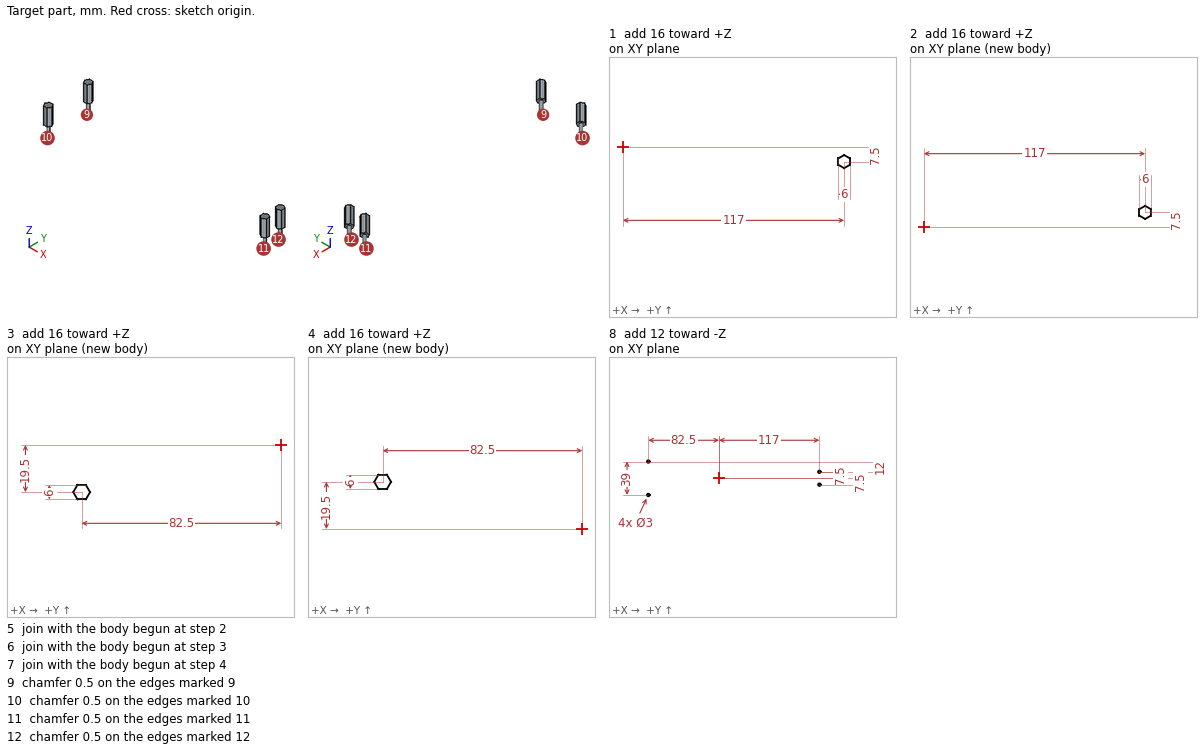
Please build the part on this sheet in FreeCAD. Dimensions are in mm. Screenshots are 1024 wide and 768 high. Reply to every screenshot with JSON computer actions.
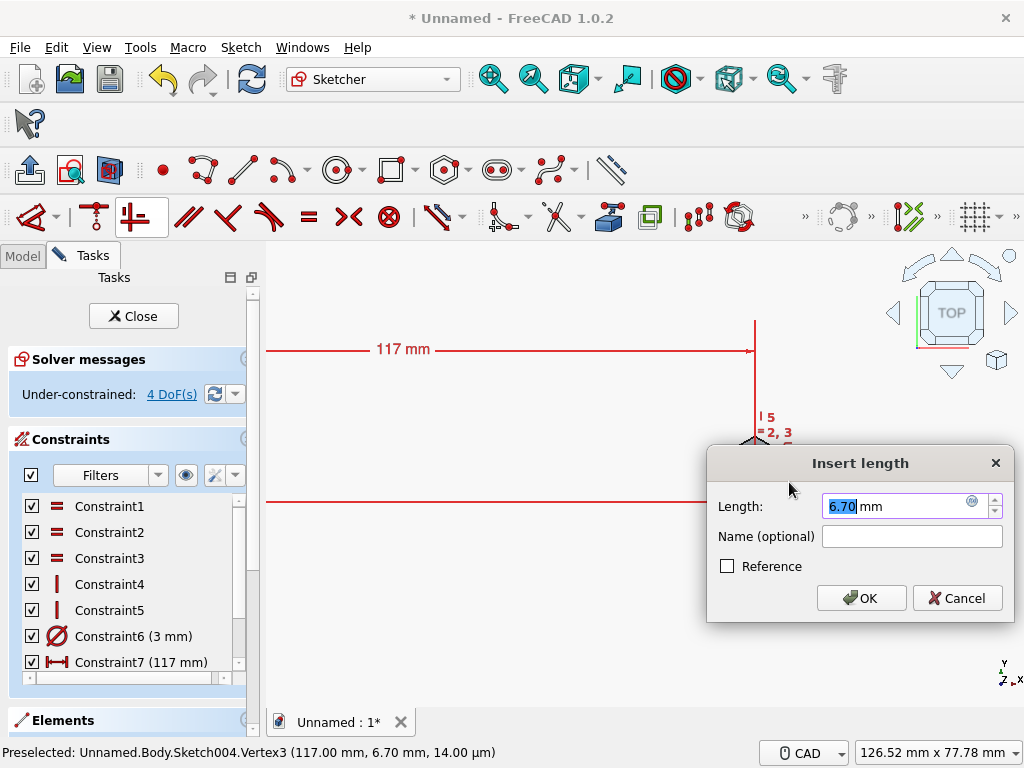
{"action": "type", "text": "7.5"}
{"action": "key", "text": "Return"}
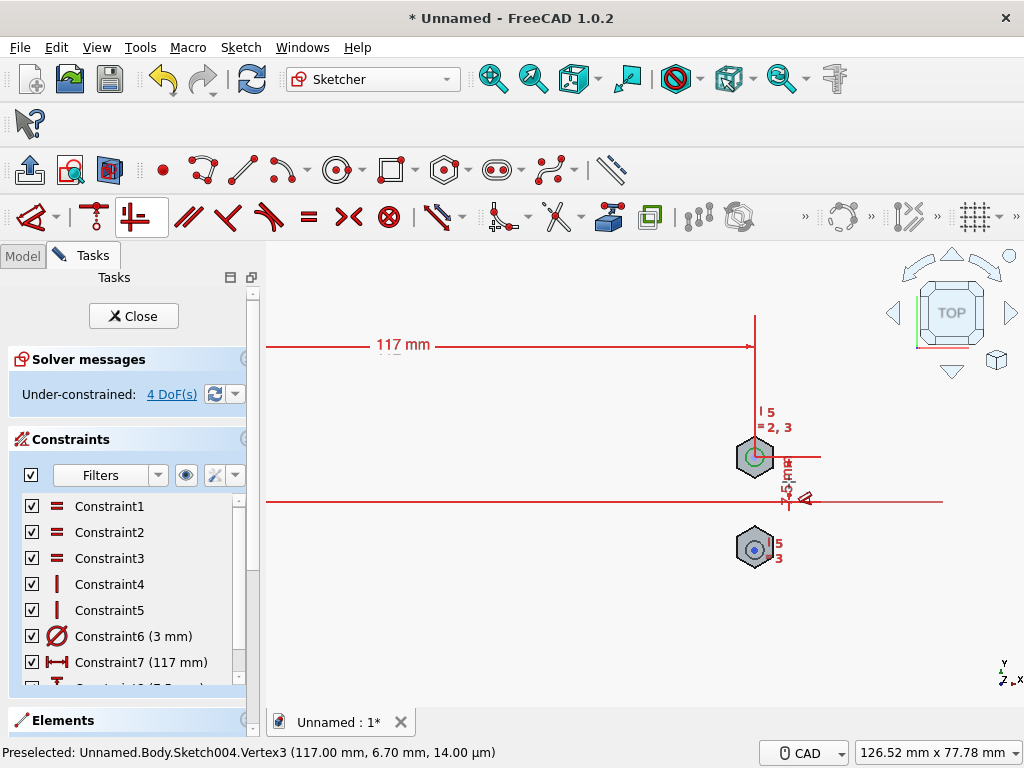
{"action": "left_click", "coordinate": [755, 550]}
{"action": "left_click", "coordinate": [789, 526]}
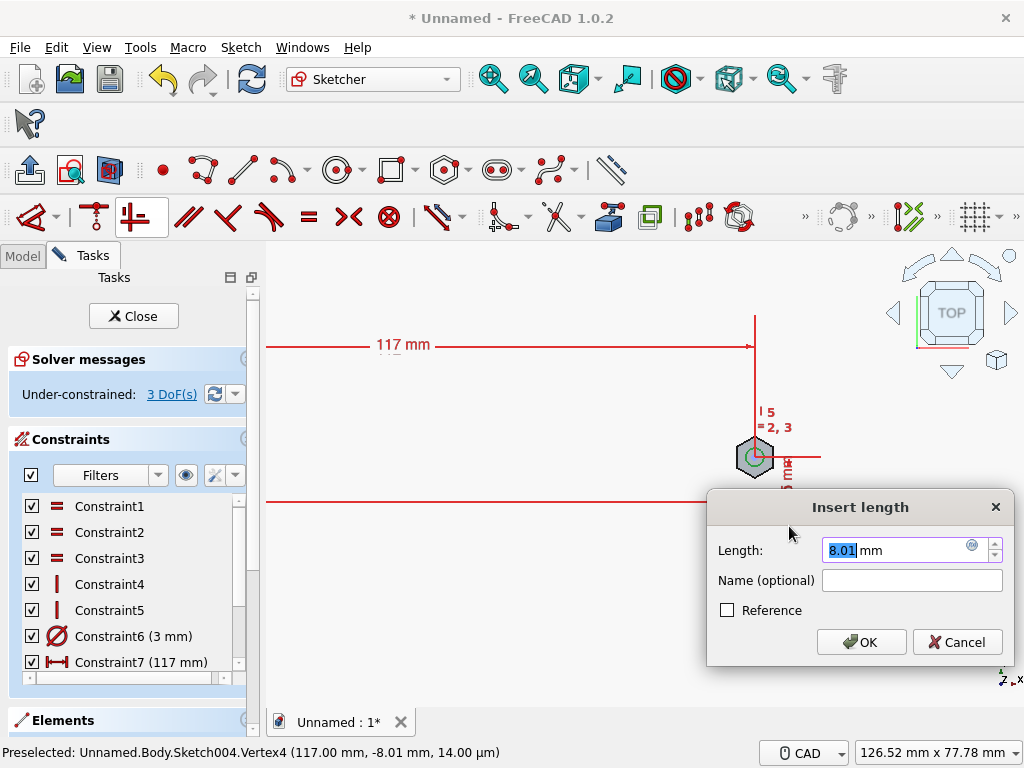
{"action": "type", "text": "7.5"}
{"action": "key", "text": "Return"}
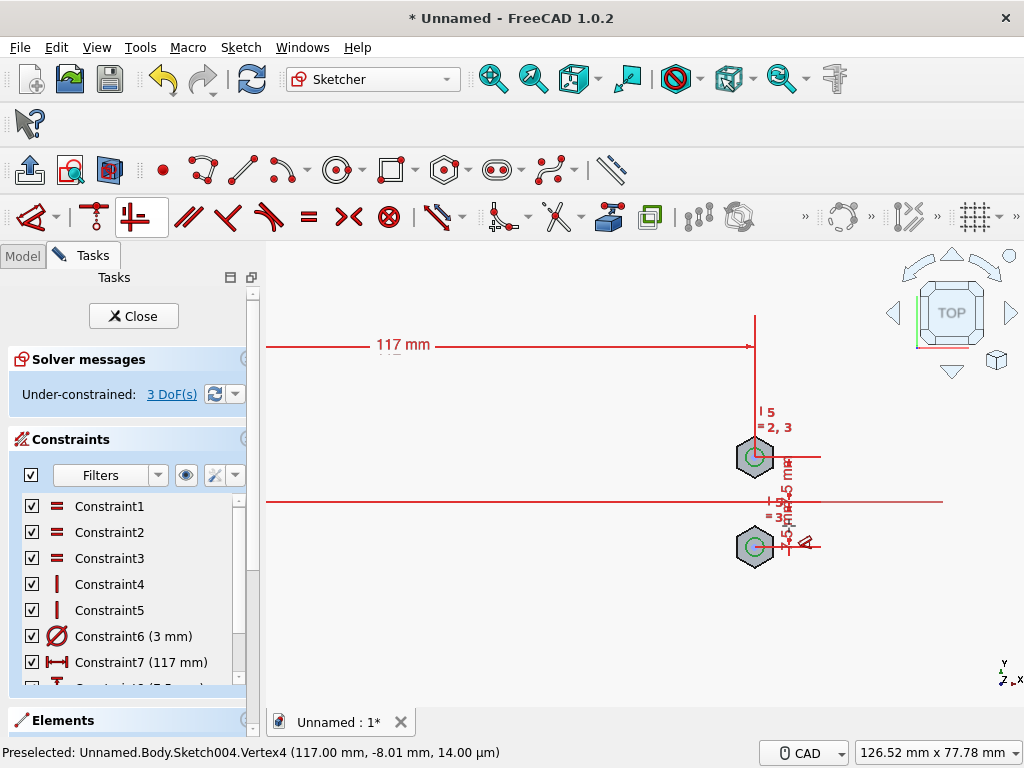
{"action": "scroll", "coordinate": [757, 462], "scroll_direction": "down", "scroll_amount": 6}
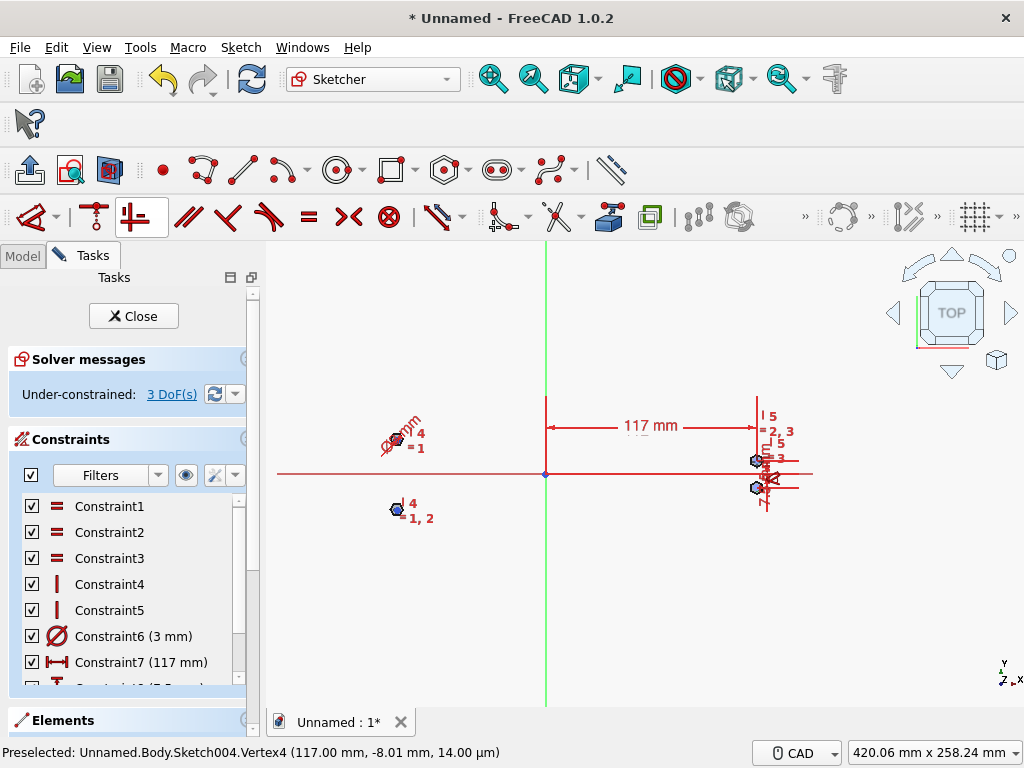
{"action": "left_click", "coordinate": [397, 440]}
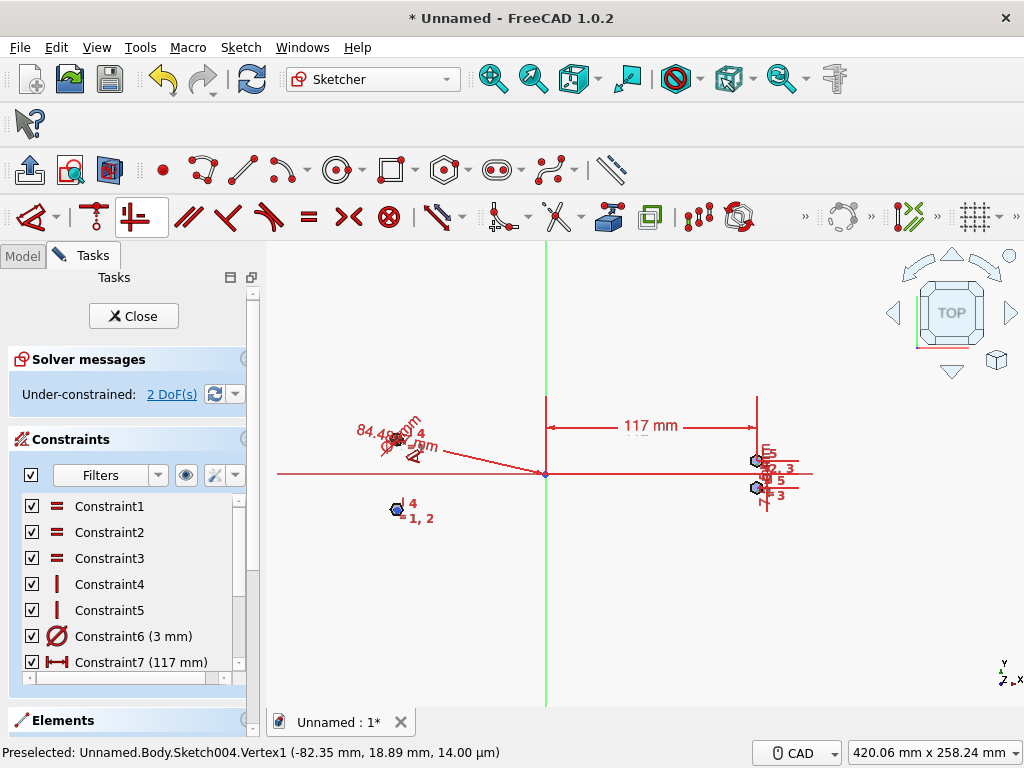
{"action": "left_click", "coordinate": [397, 510]}
{"action": "left_click", "coordinate": [363, 459]}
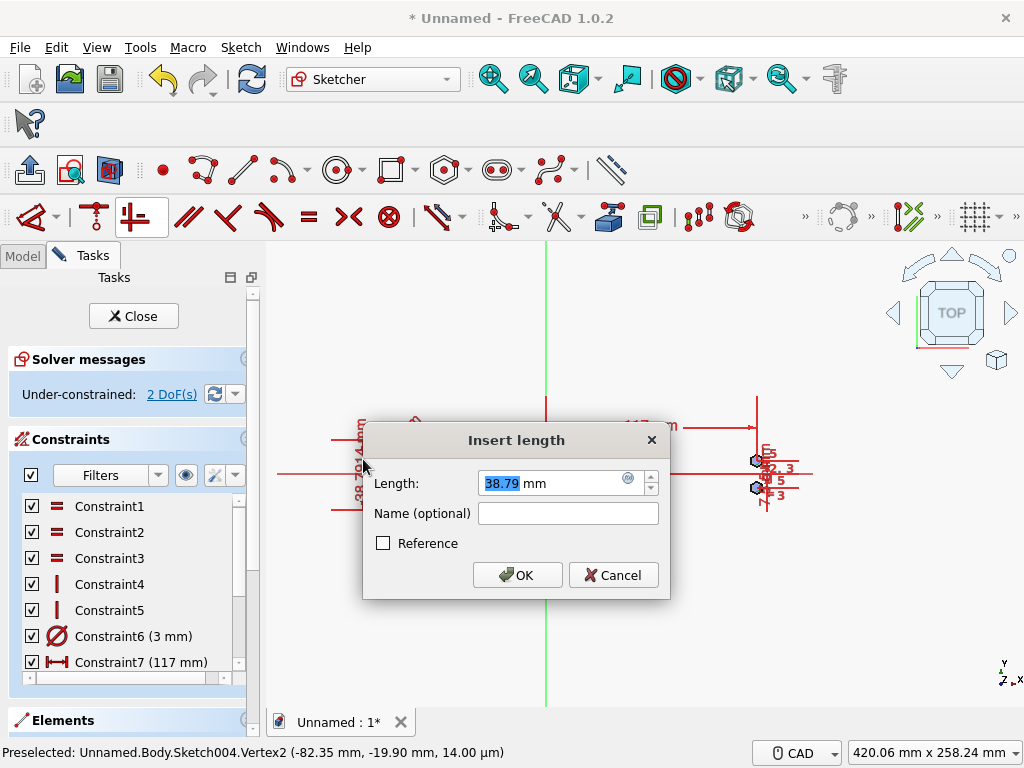
{"action": "type", "text": "39"}
{"action": "key", "text": "Return"}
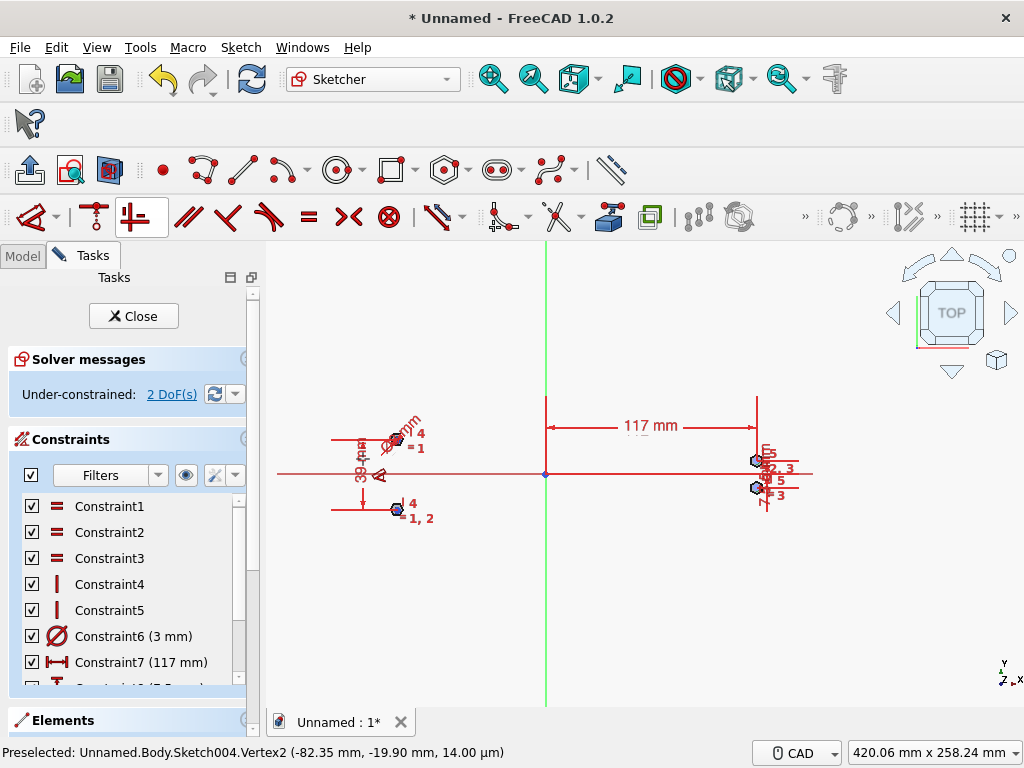
{"action": "scroll", "coordinate": [397, 440], "scroll_direction": "up", "scroll_amount": 4}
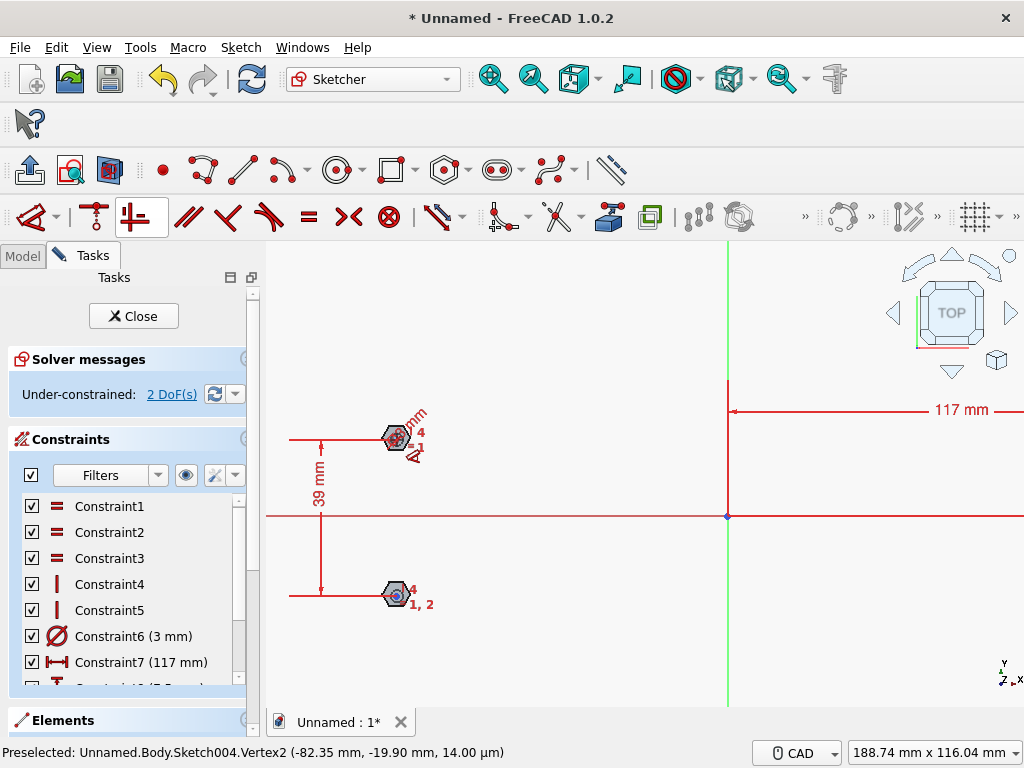
{"action": "left_click", "coordinate": [397, 440]}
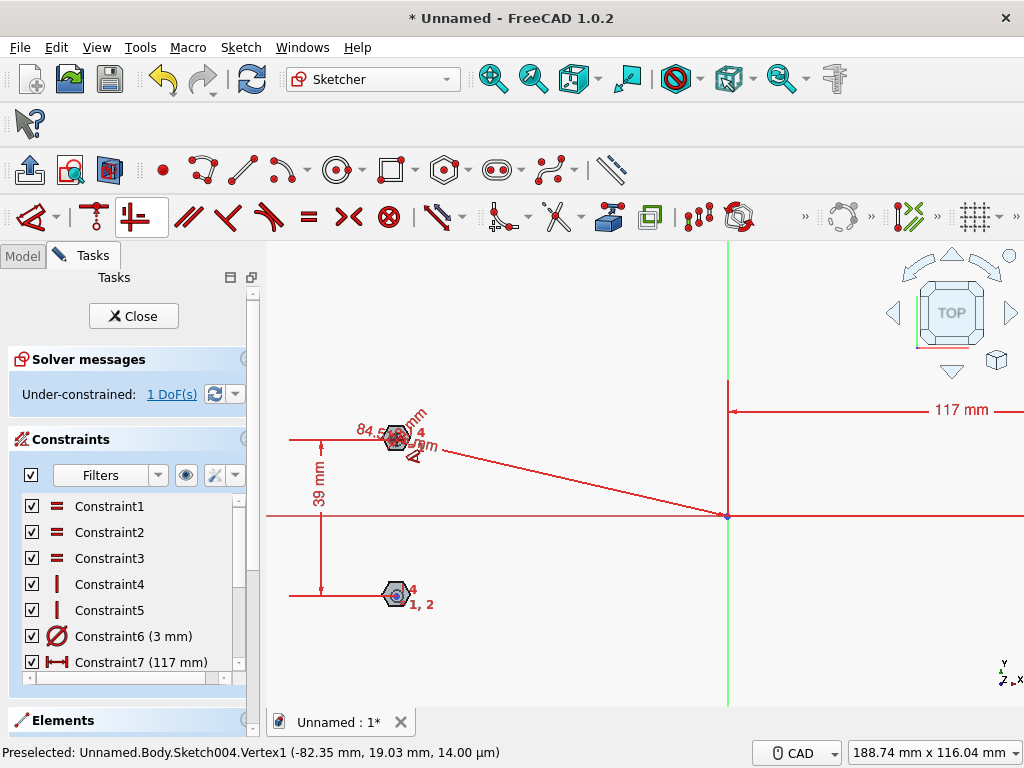
{"action": "scroll", "coordinate": [397, 440], "scroll_direction": "down", "scroll_amount": 4}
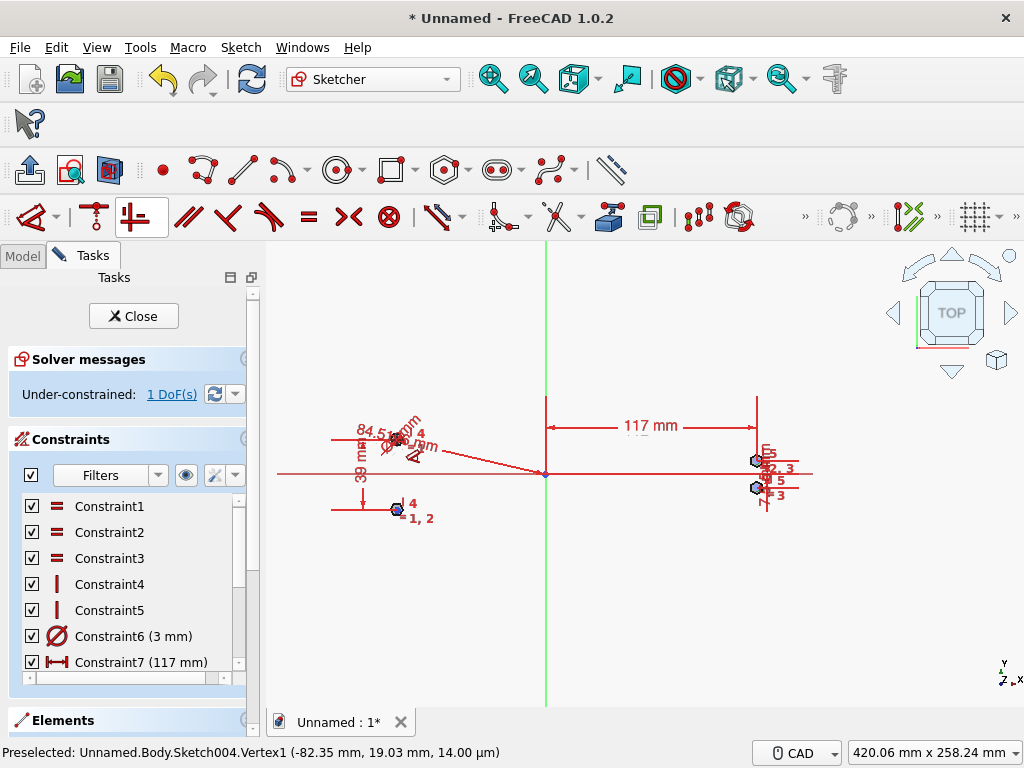
{"action": "scroll", "coordinate": [757, 461], "scroll_direction": "up", "scroll_amount": 4}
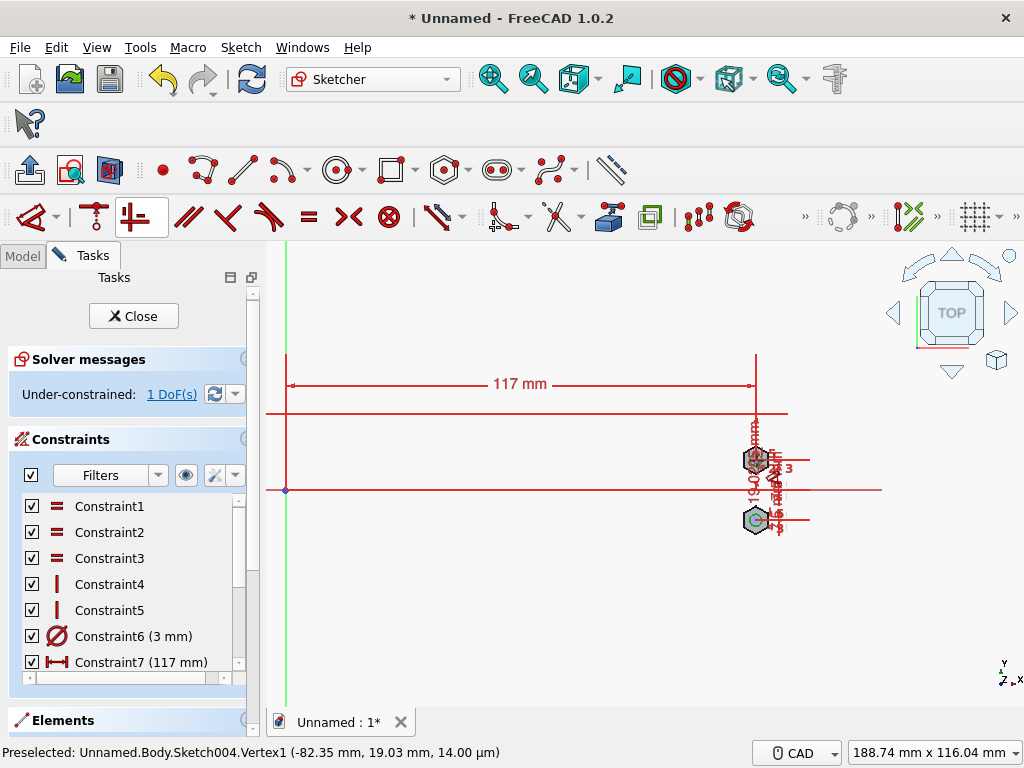
{"action": "left_click", "coordinate": [756, 460]}
{"action": "left_click", "coordinate": [790, 437]}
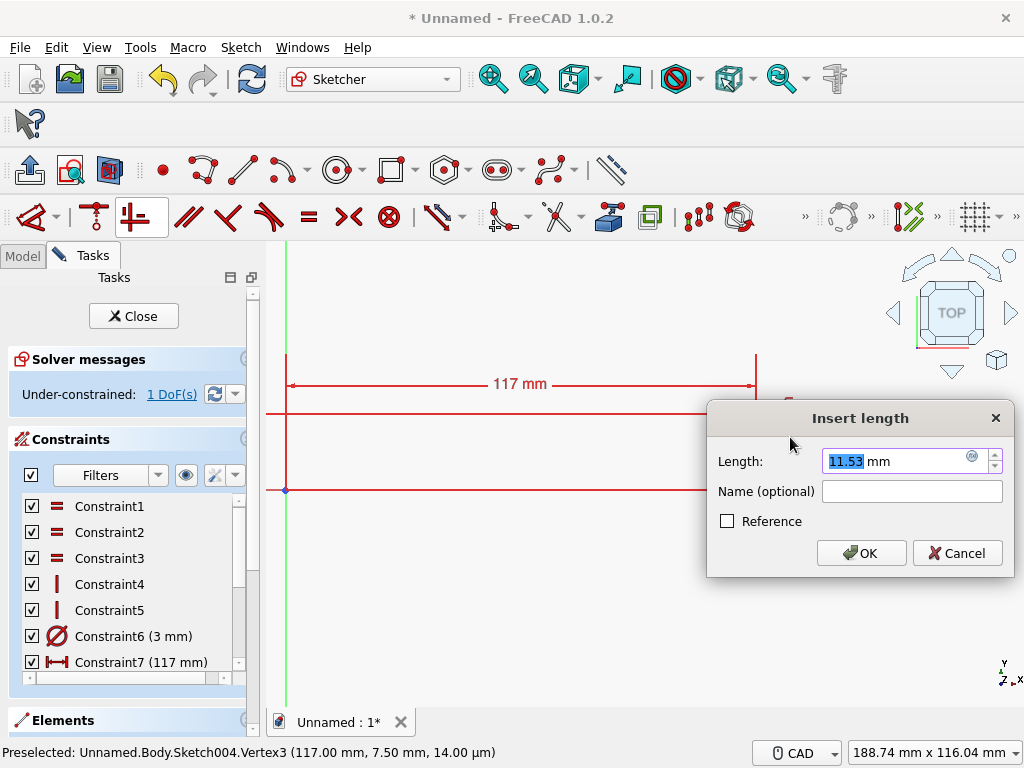
{"action": "type", "text": "12"}
{"action": "key", "text": "Return"}